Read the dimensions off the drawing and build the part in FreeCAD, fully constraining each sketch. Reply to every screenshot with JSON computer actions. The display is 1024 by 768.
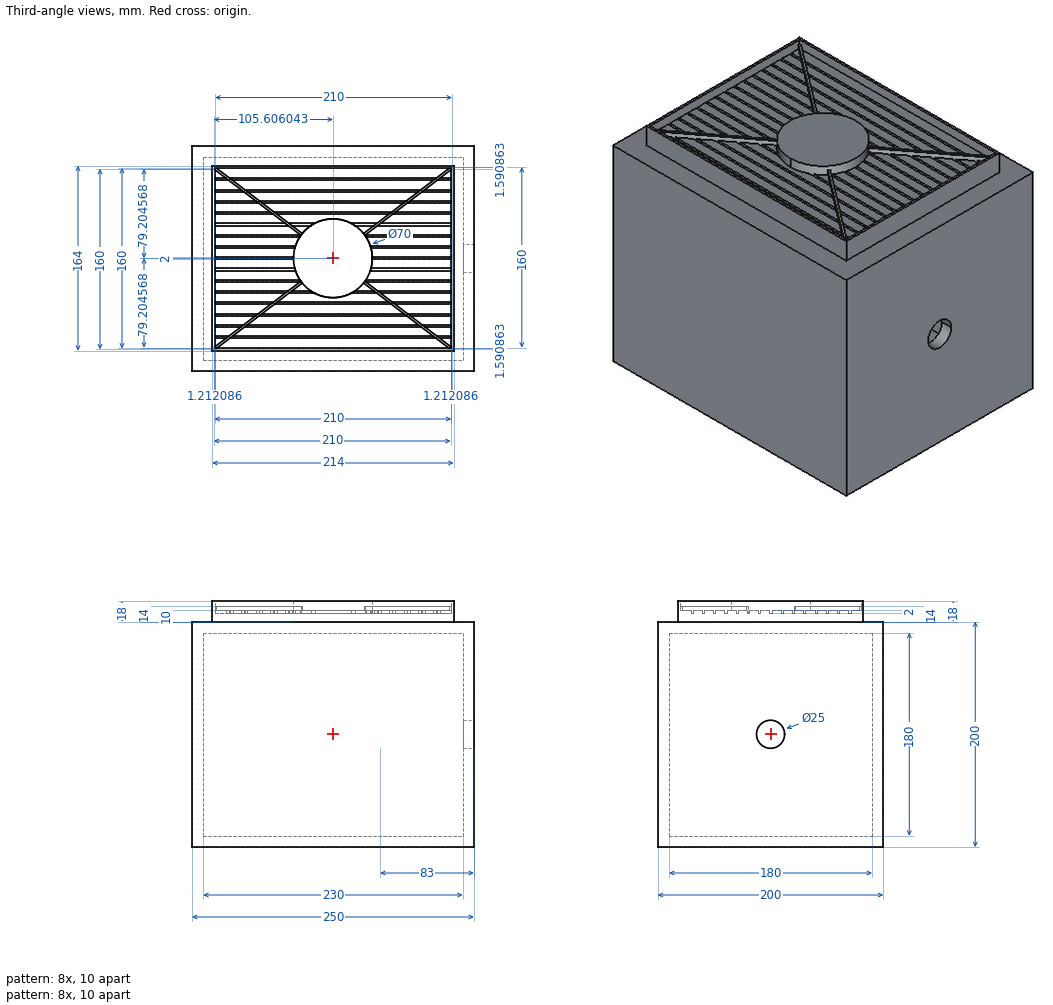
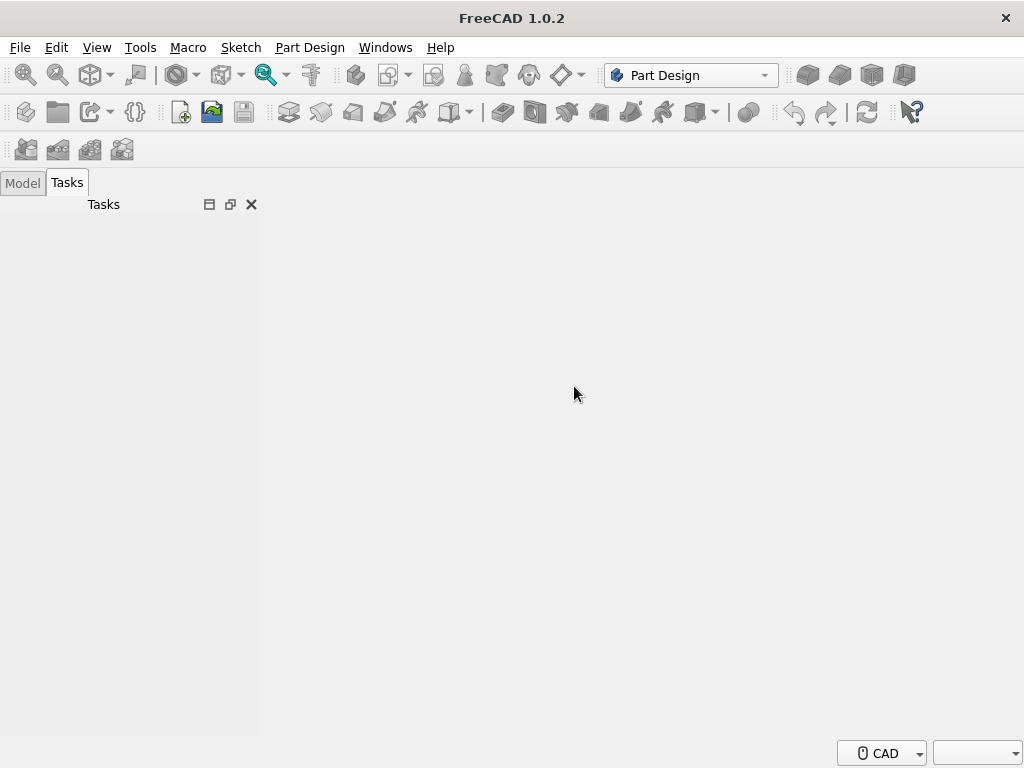
{"action": "left_click", "coordinate": [180, 112]}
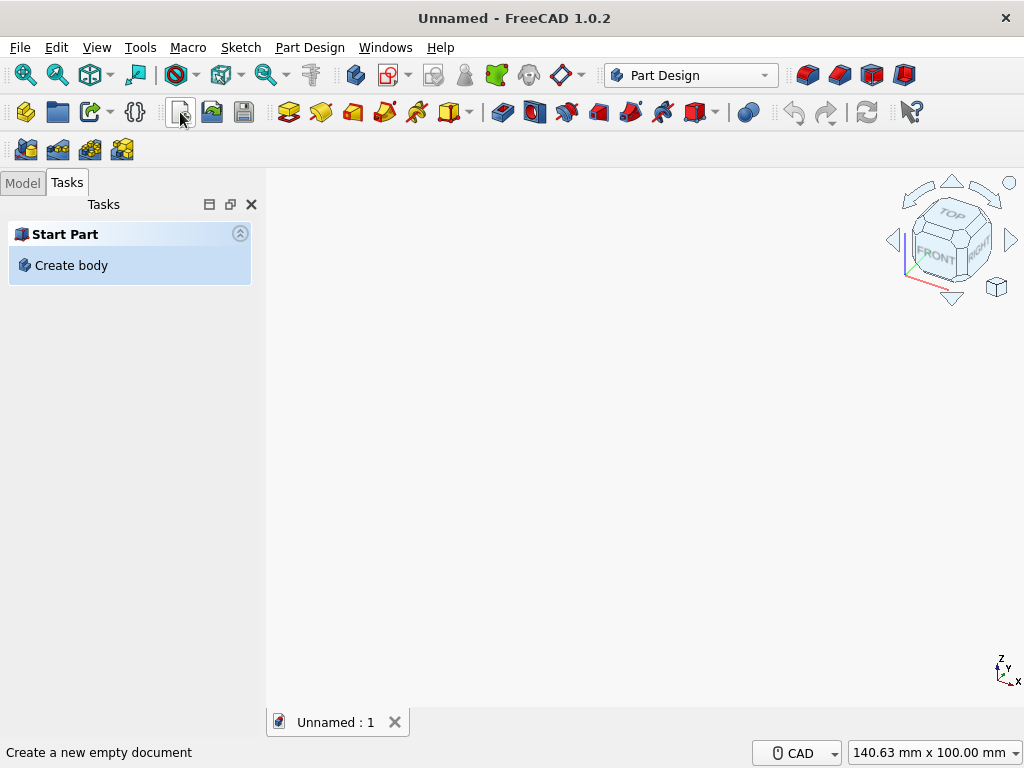
{"action": "left_click", "coordinate": [388, 76]}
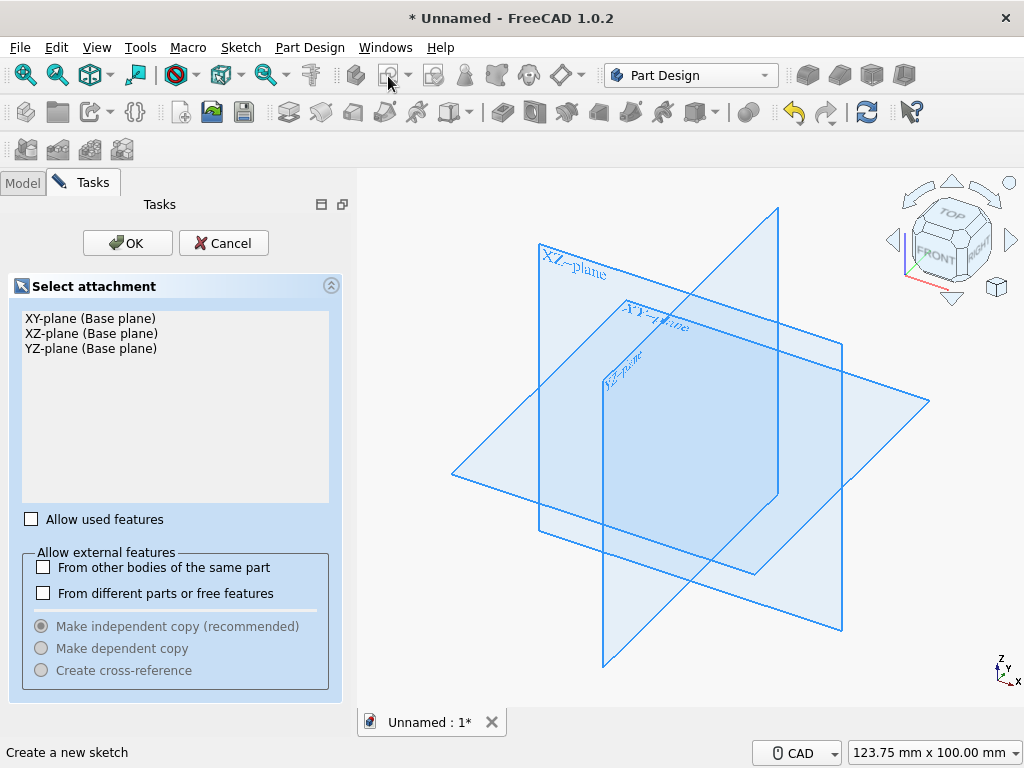
{"action": "left_click", "coordinate": [82, 348]}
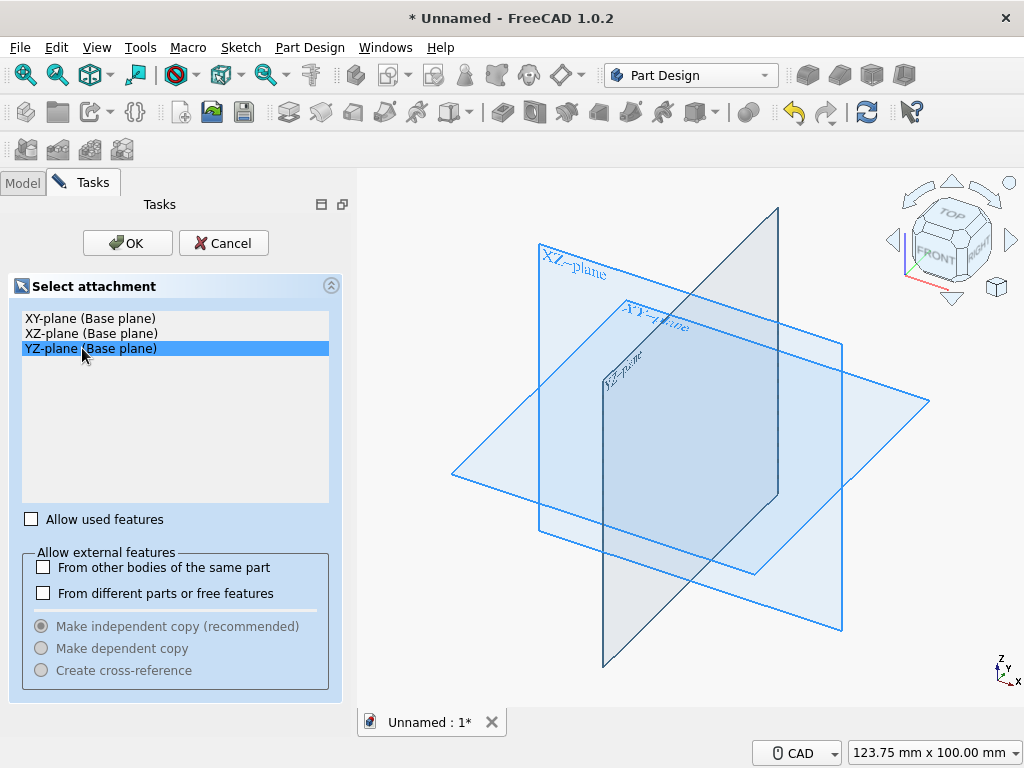
{"action": "left_click", "coordinate": [128, 243]}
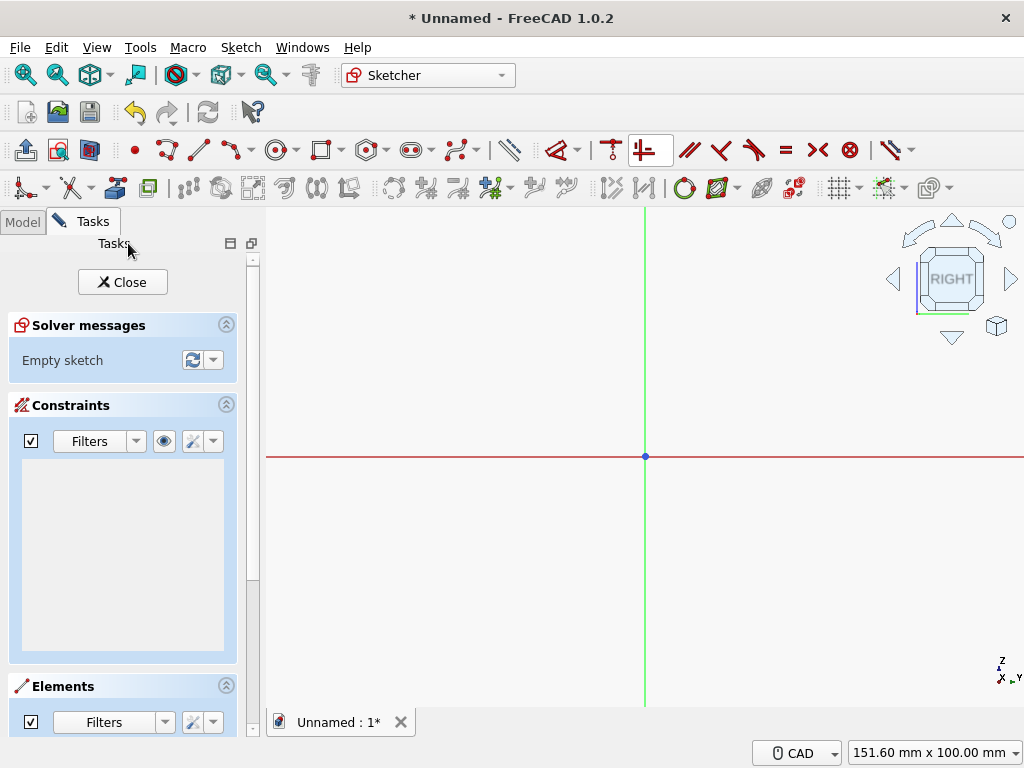
{"action": "scroll", "coordinate": [547, 457], "scroll_direction": "down", "scroll_amount": 6}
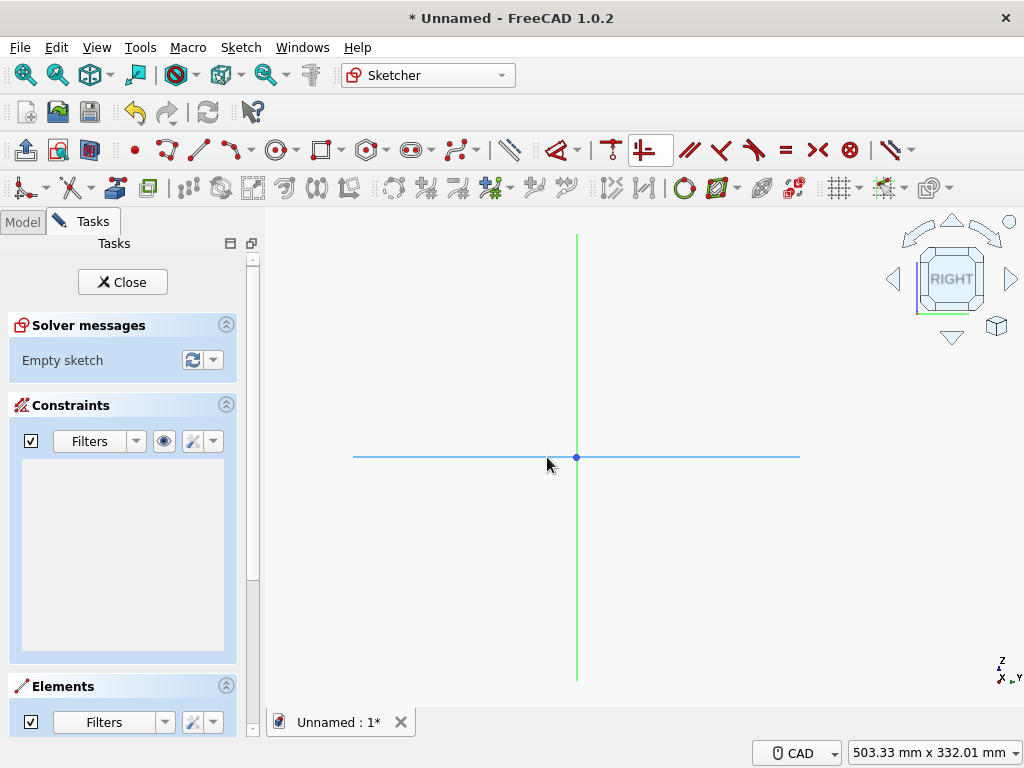
{"action": "left_click", "coordinate": [344, 150]}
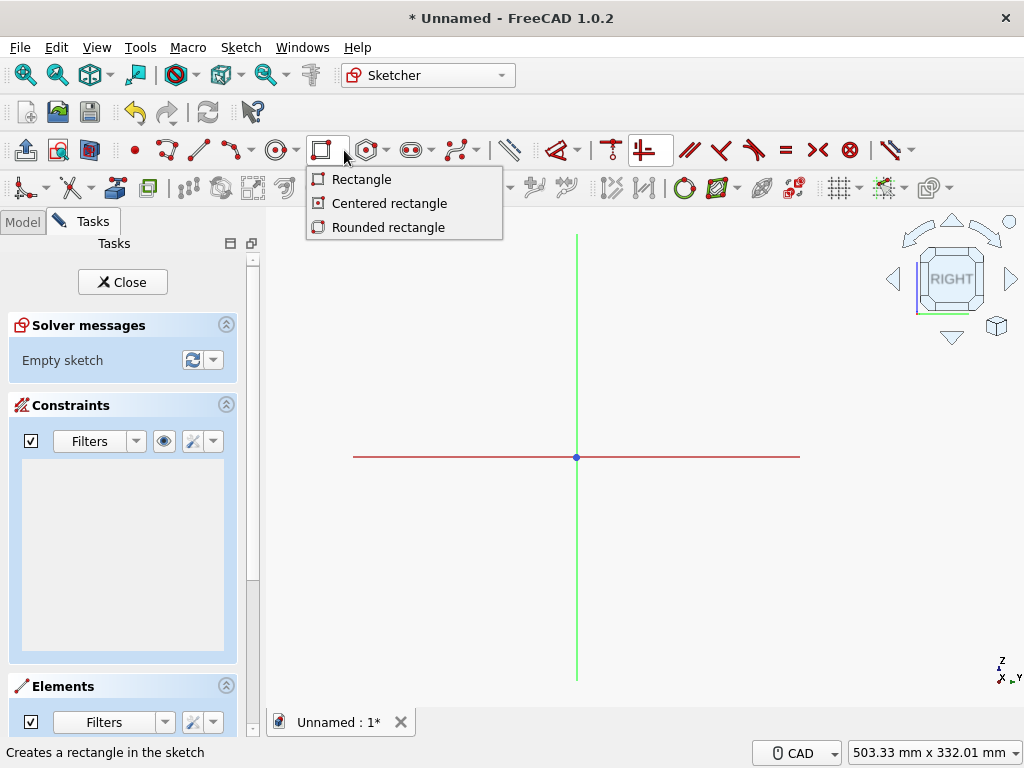
{"action": "left_click", "coordinate": [404, 203]}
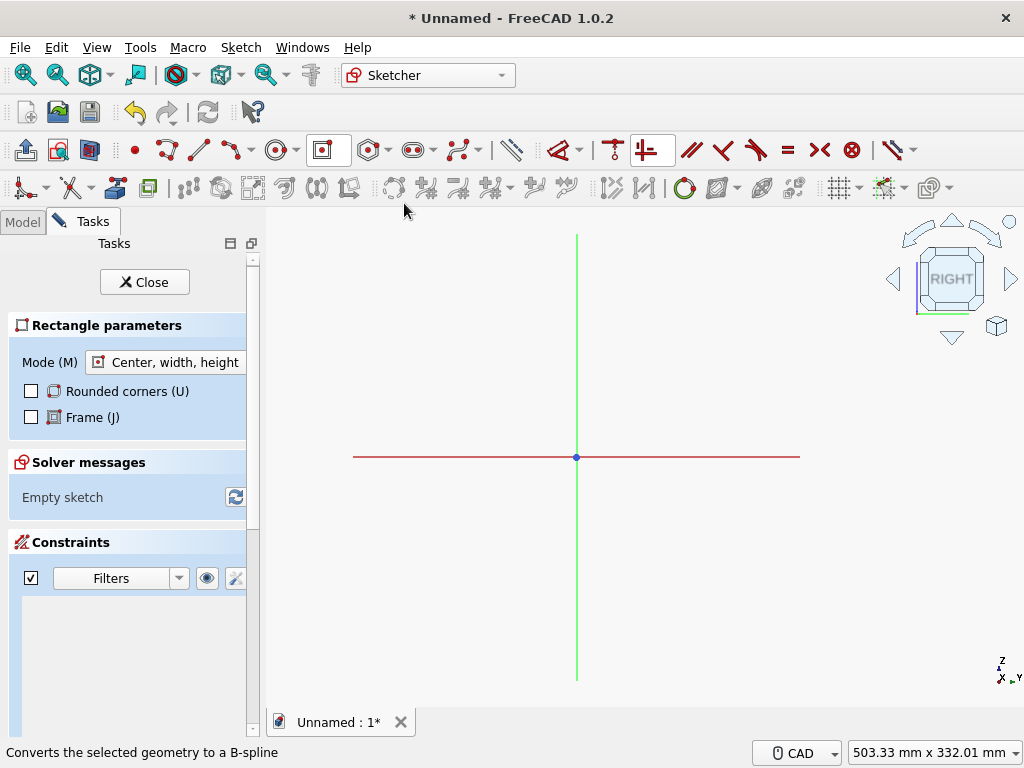
{"action": "left_click", "coordinate": [577, 457]}
{"action": "left_click", "coordinate": [727, 307]}
{"action": "key", "text": "Escape"}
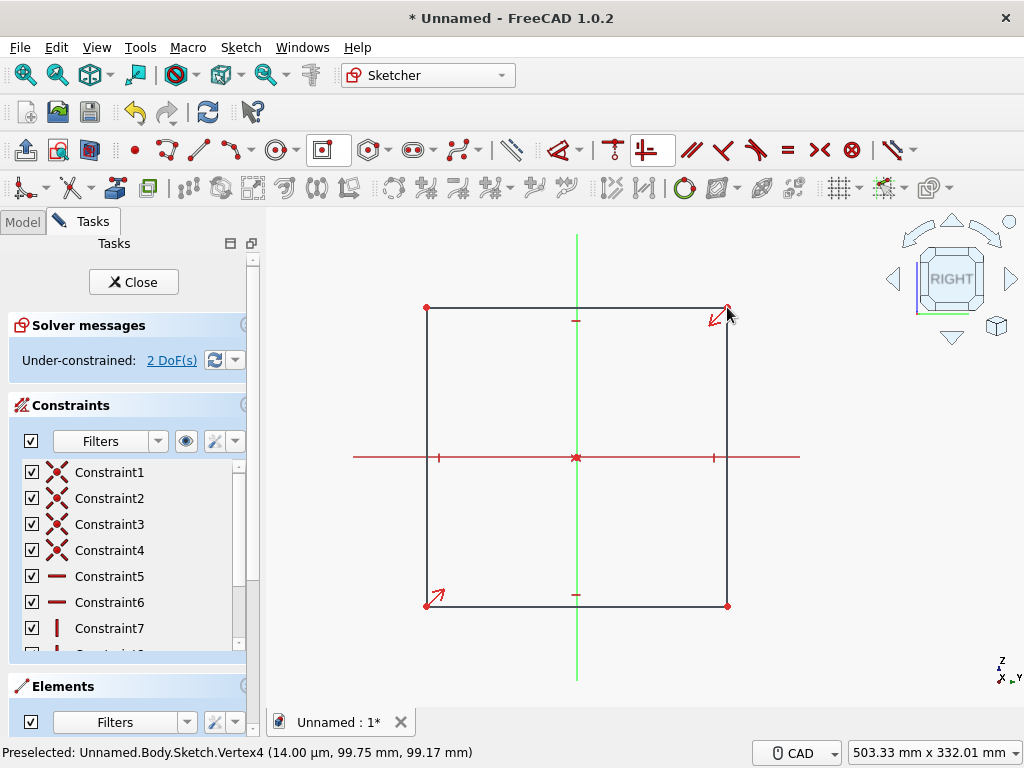
{"action": "left_click", "coordinate": [558, 150]}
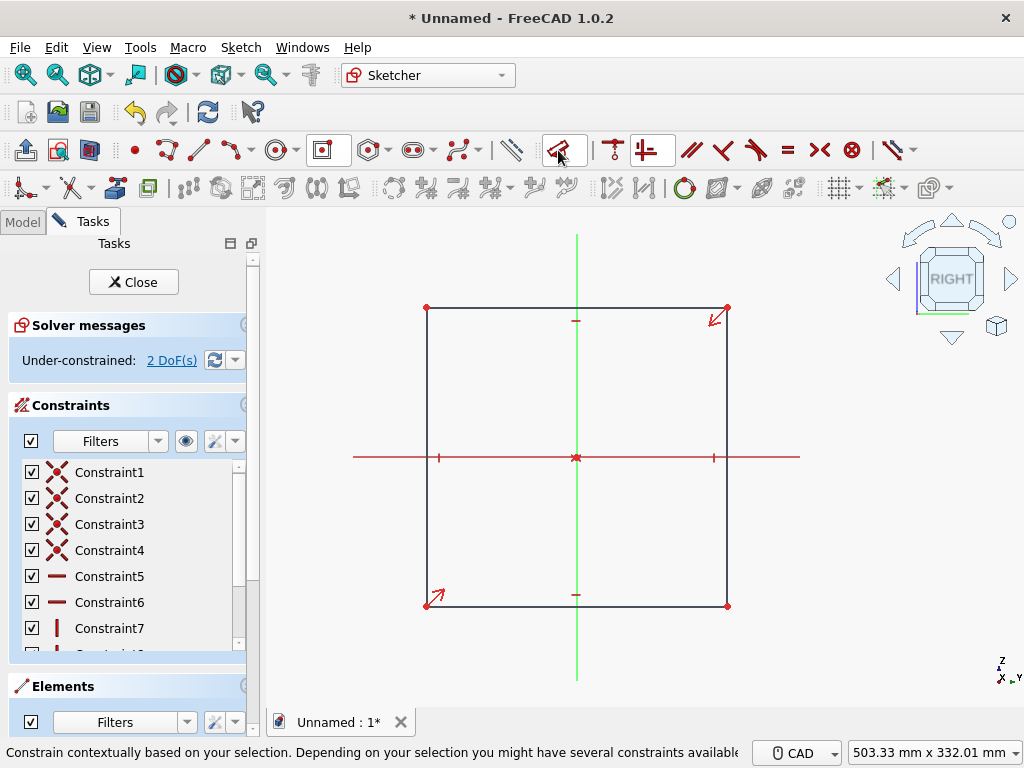
{"action": "left_click", "coordinate": [517, 607]}
{"action": "left_click", "coordinate": [508, 641]}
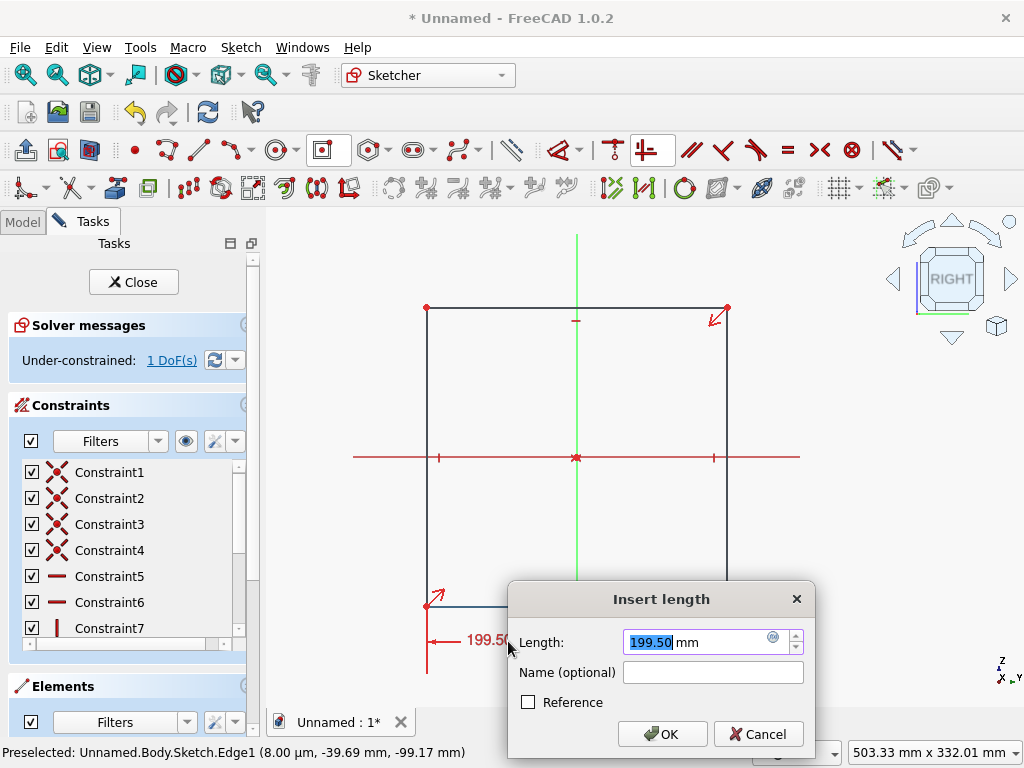
{"action": "type", "text": "200"}
{"action": "key", "text": "Return"}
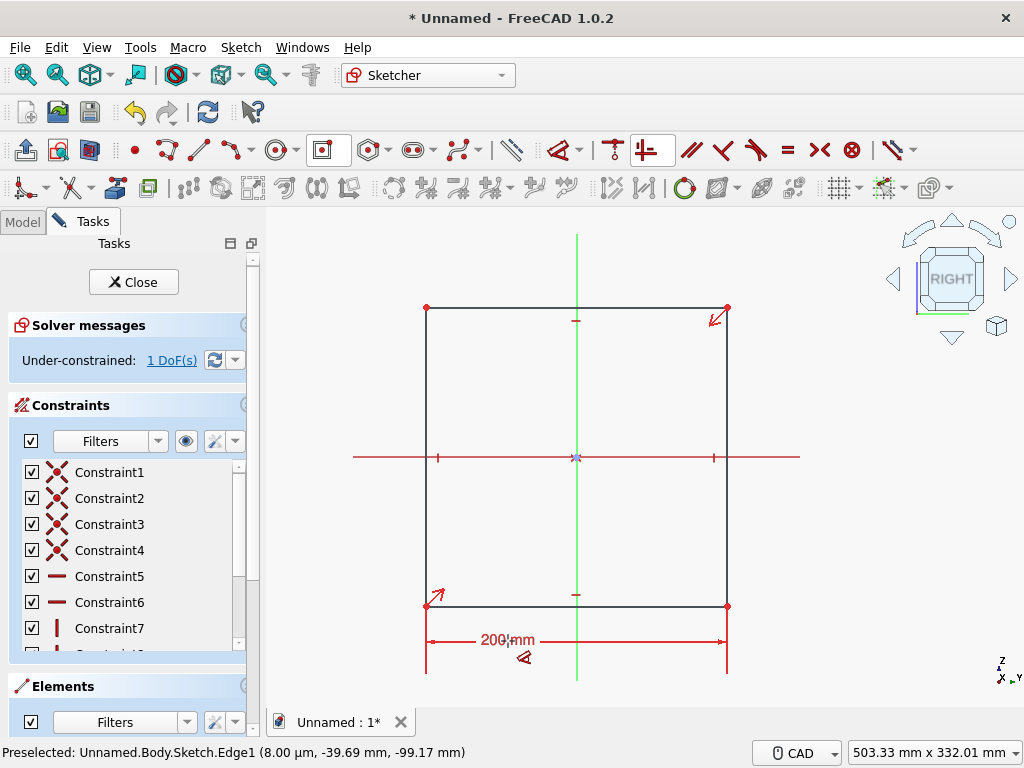
{"action": "left_click", "coordinate": [727, 517]}
{"action": "left_click", "coordinate": [761, 389]}